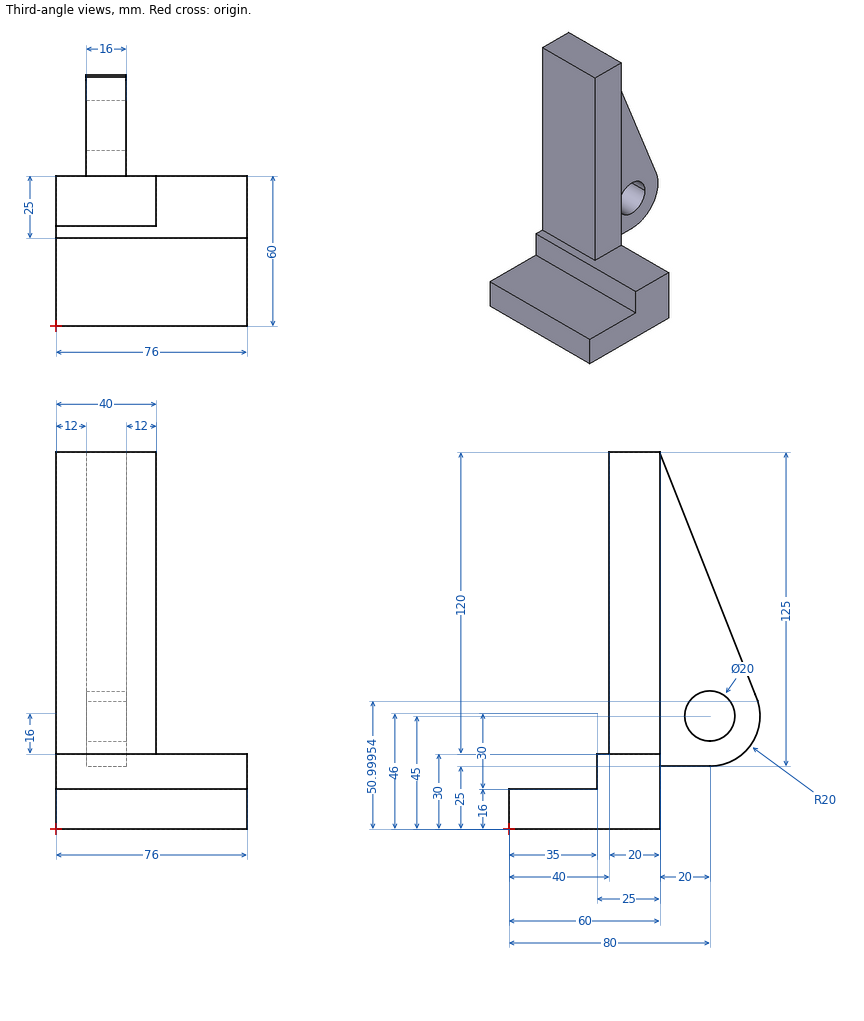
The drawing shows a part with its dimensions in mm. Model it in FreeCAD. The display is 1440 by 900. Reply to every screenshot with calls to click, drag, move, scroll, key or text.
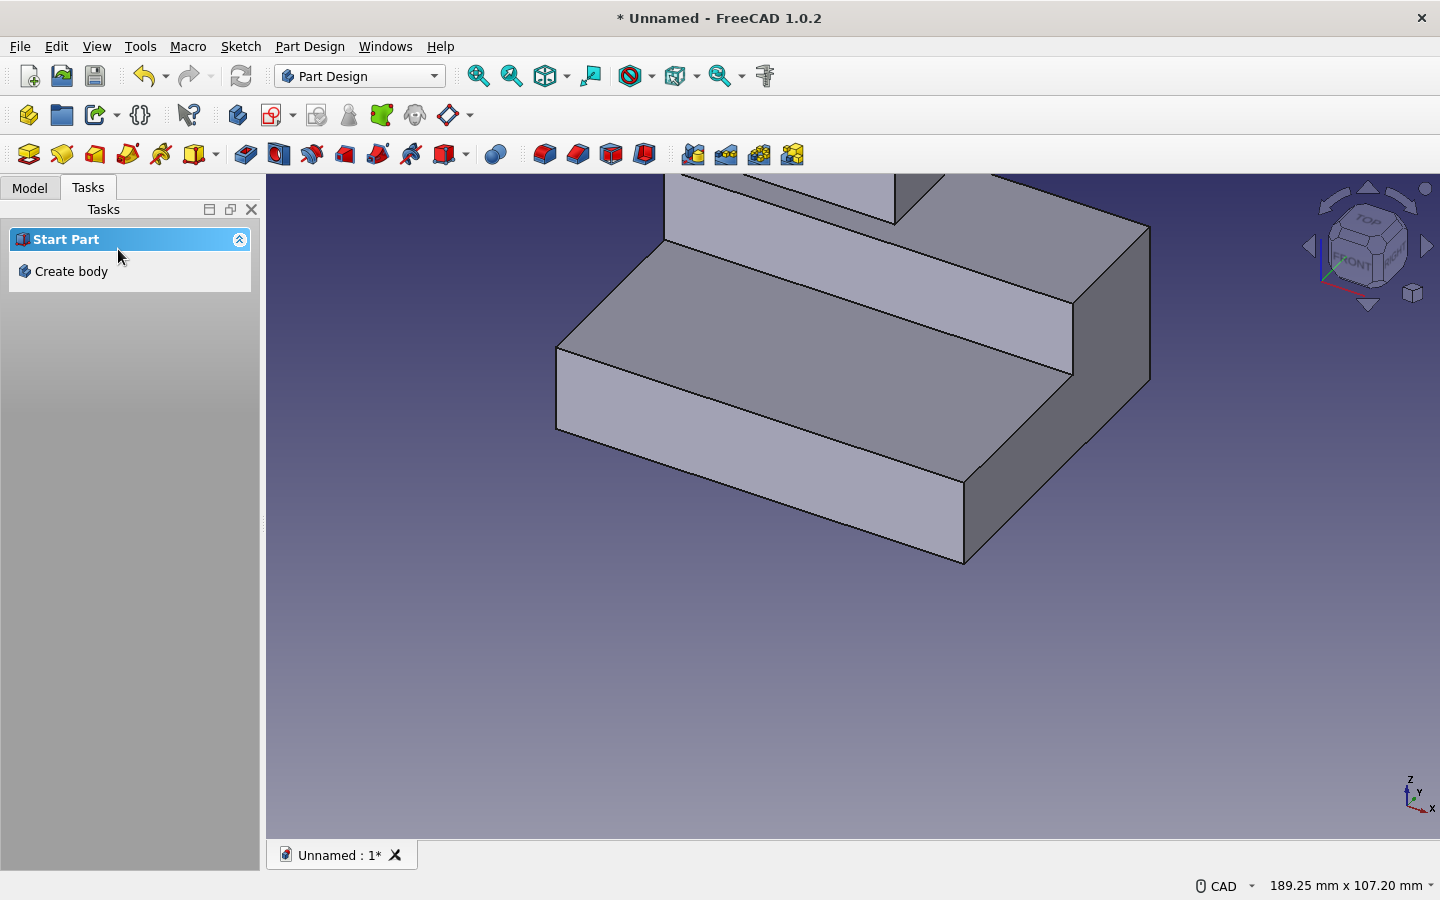
key(v)
key(f)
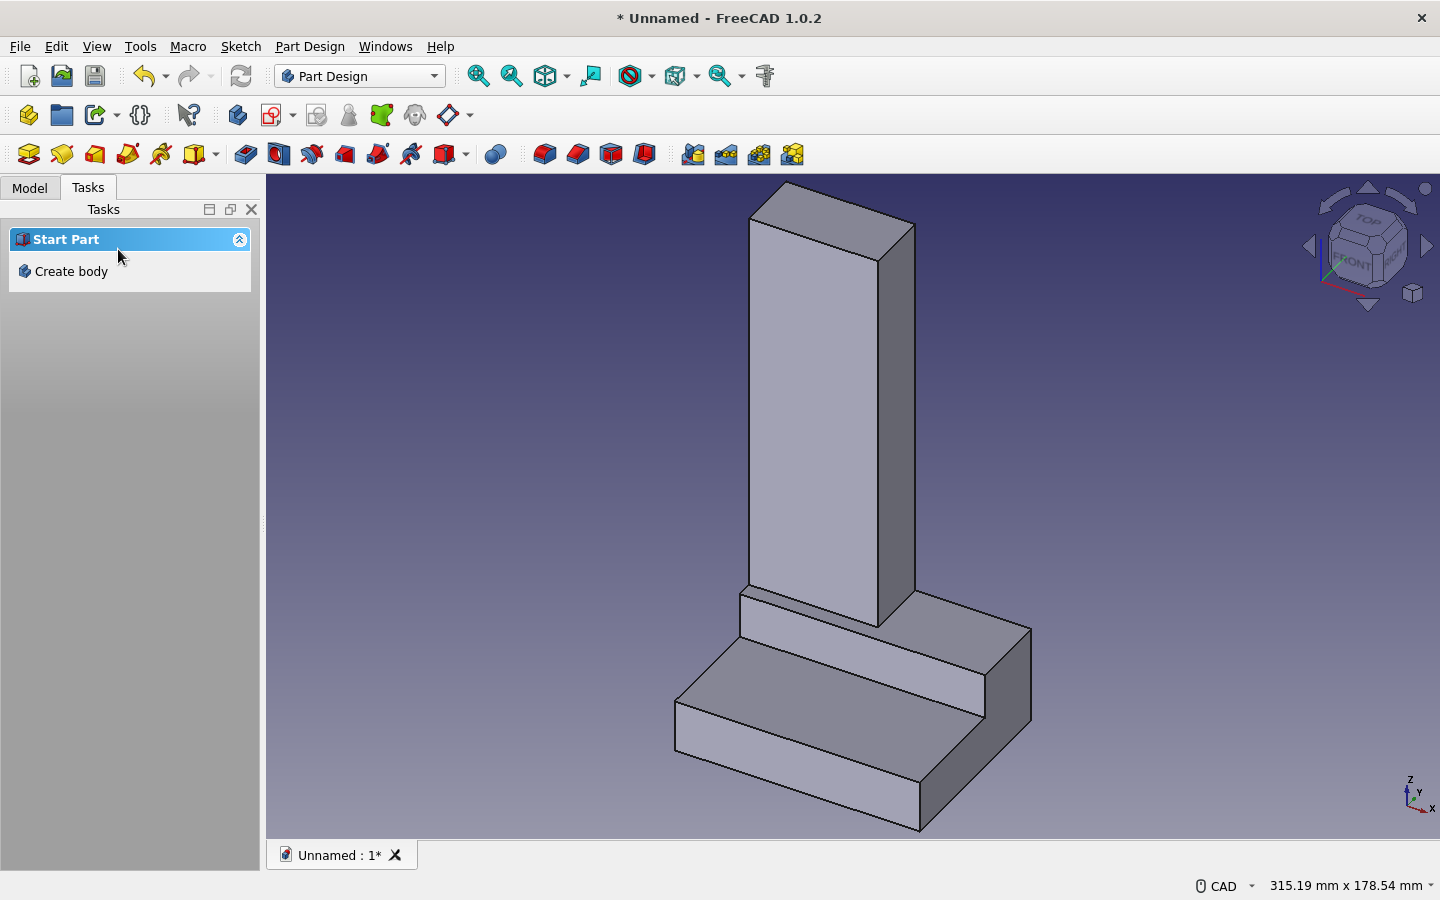
click(897, 320)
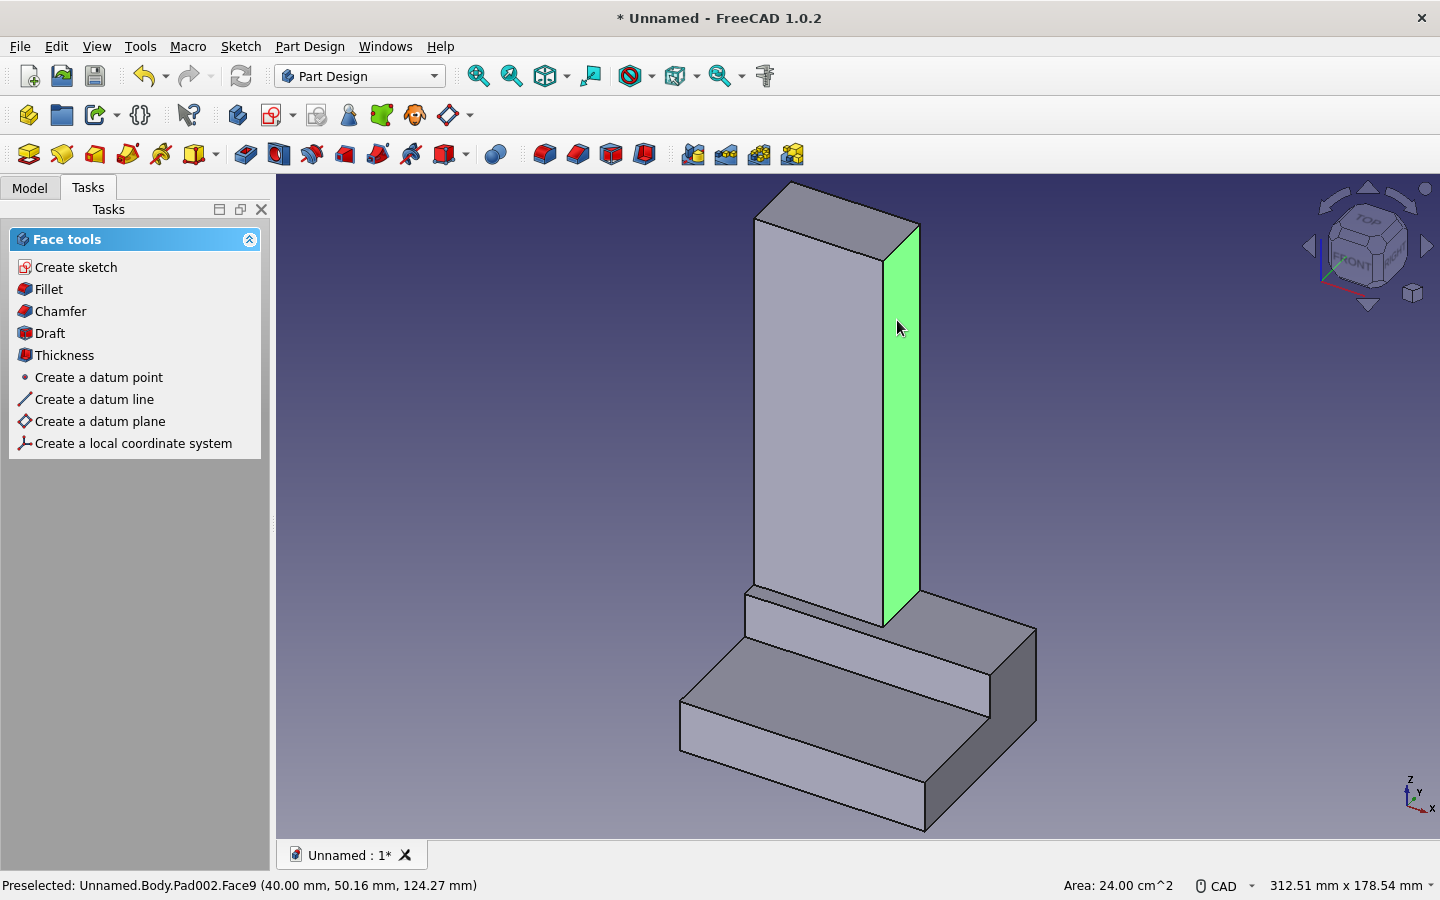
click(270, 116)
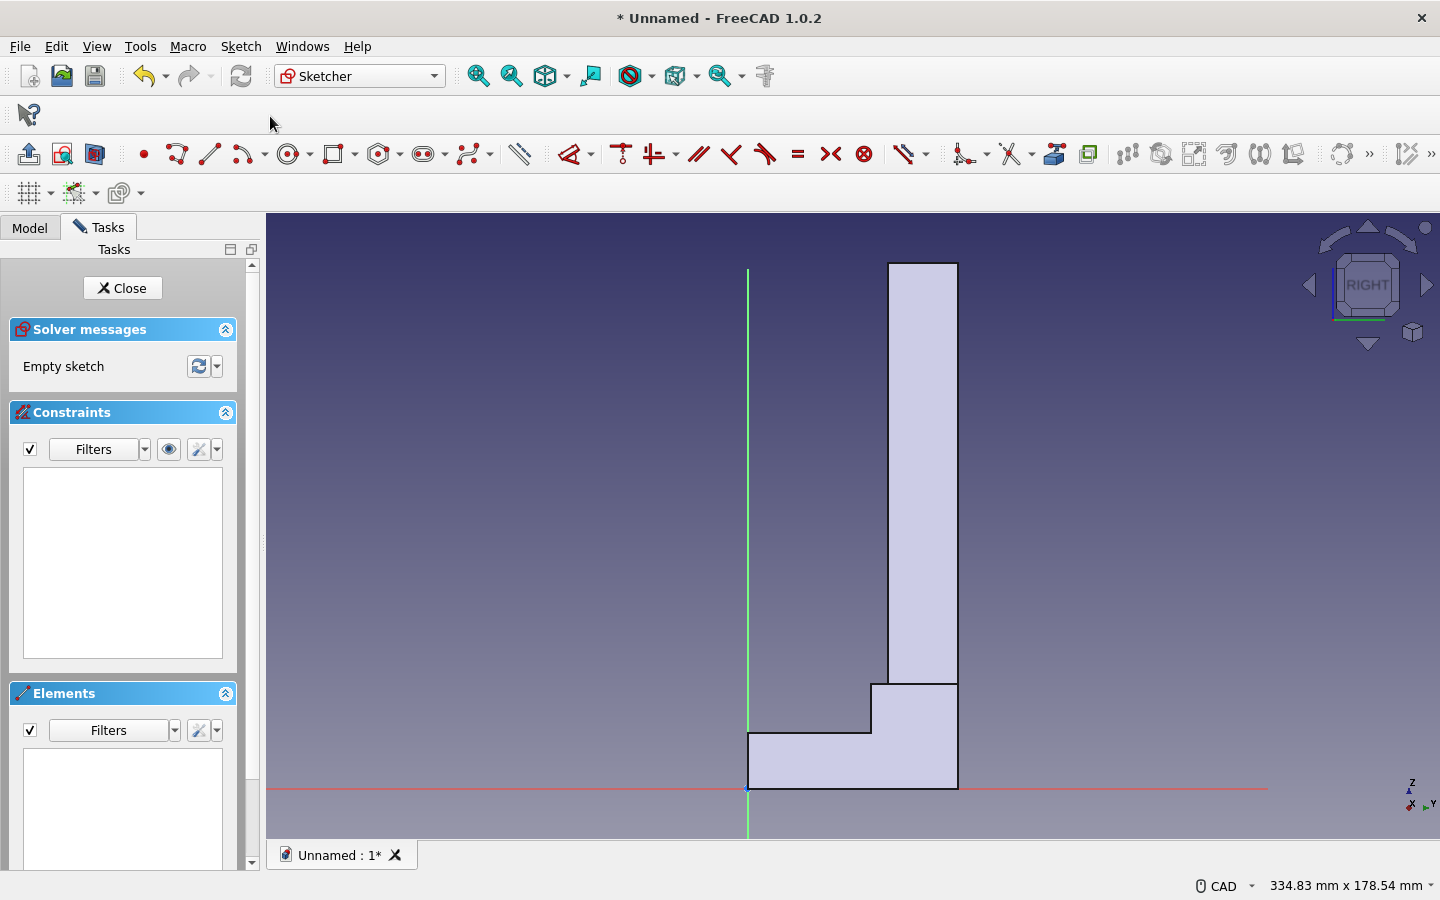
key(q)
key(s)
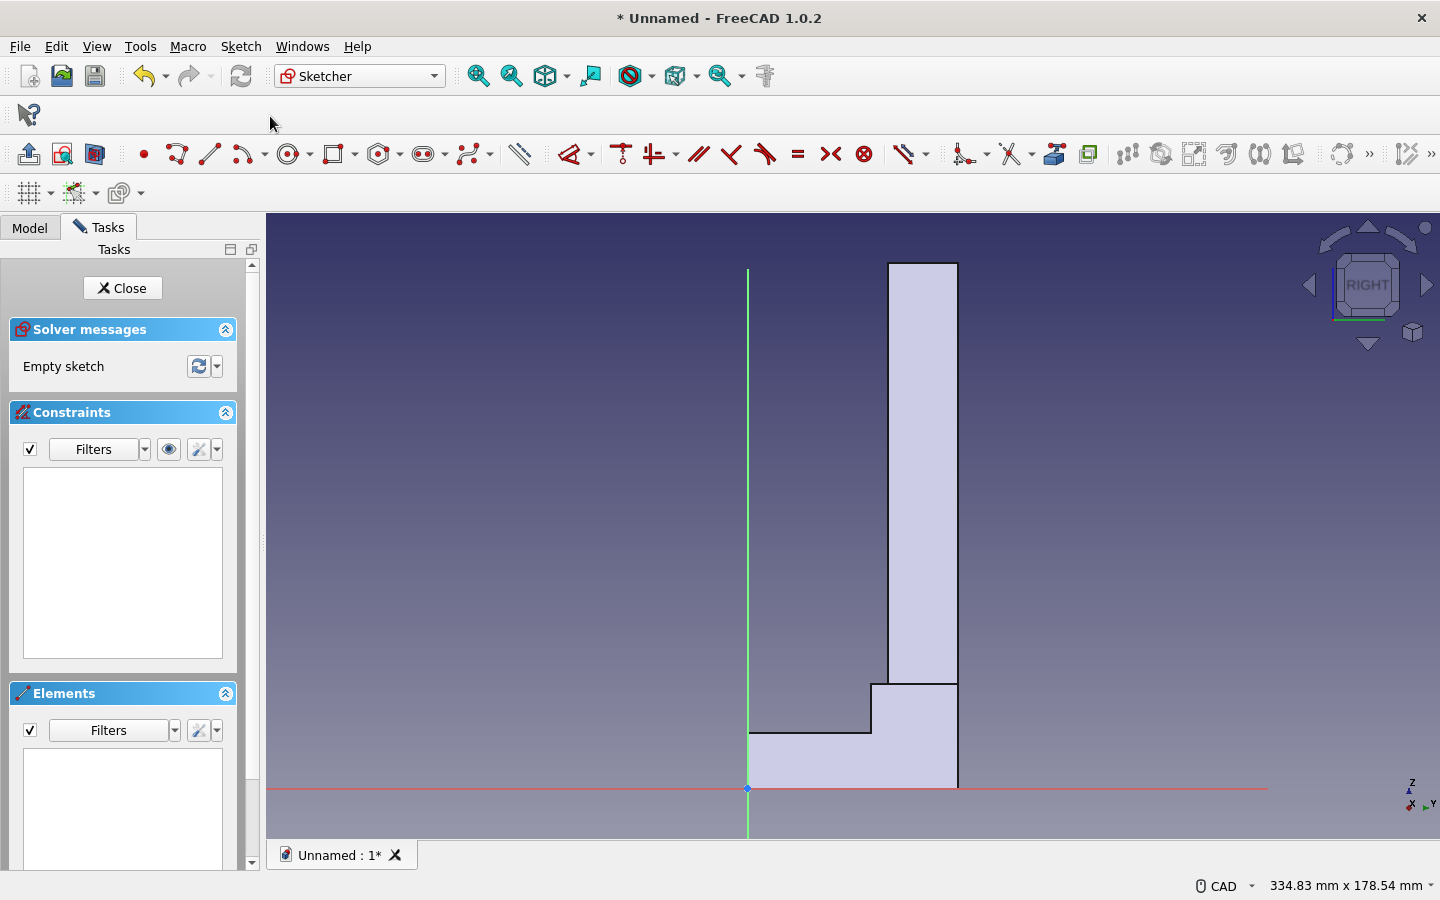
scroll(294, 526, down, 1)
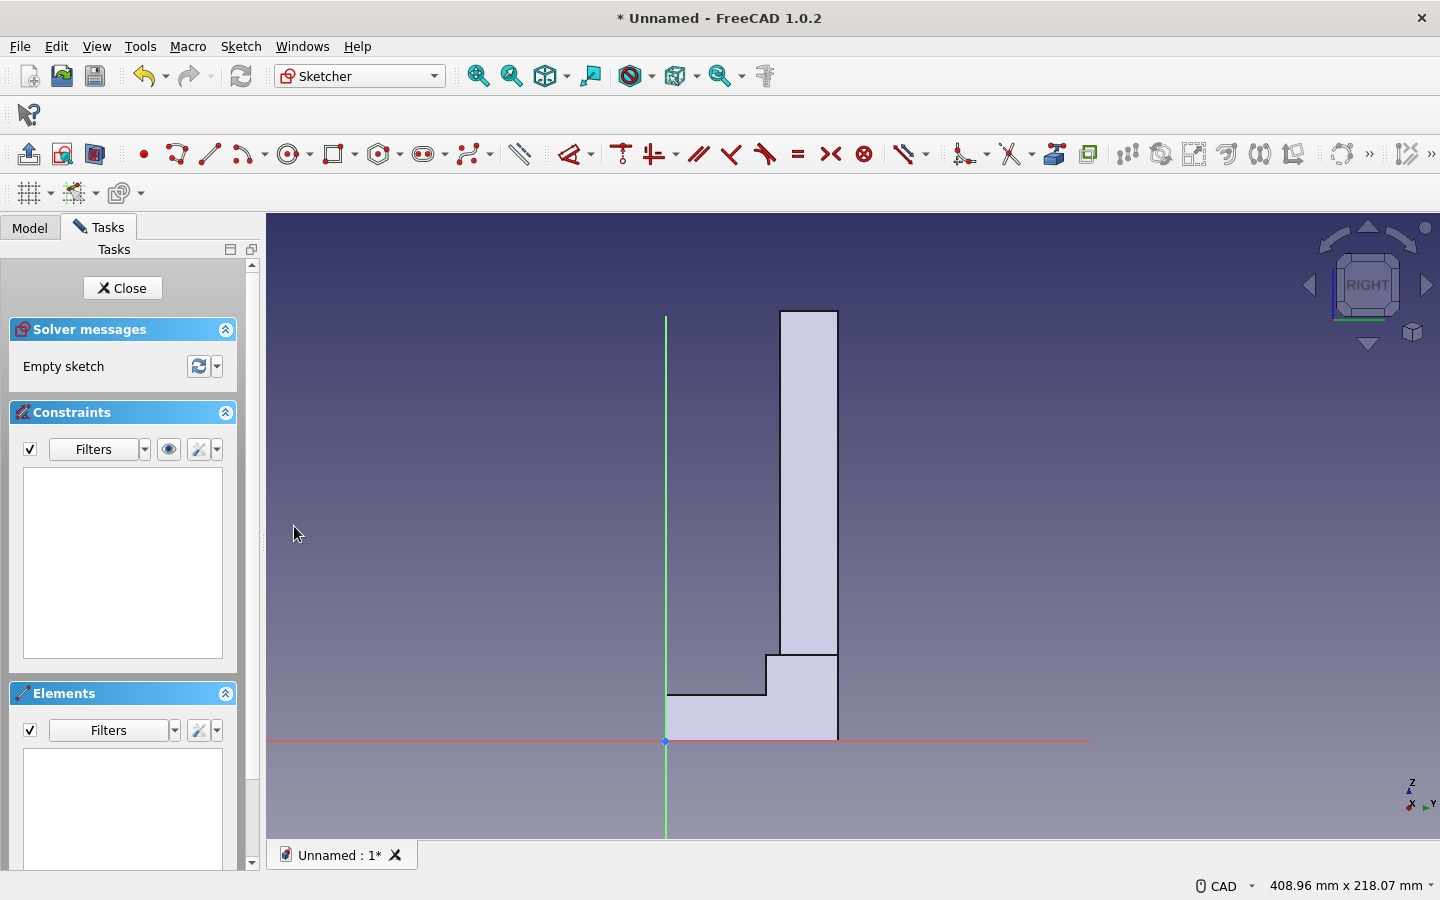
click(177, 154)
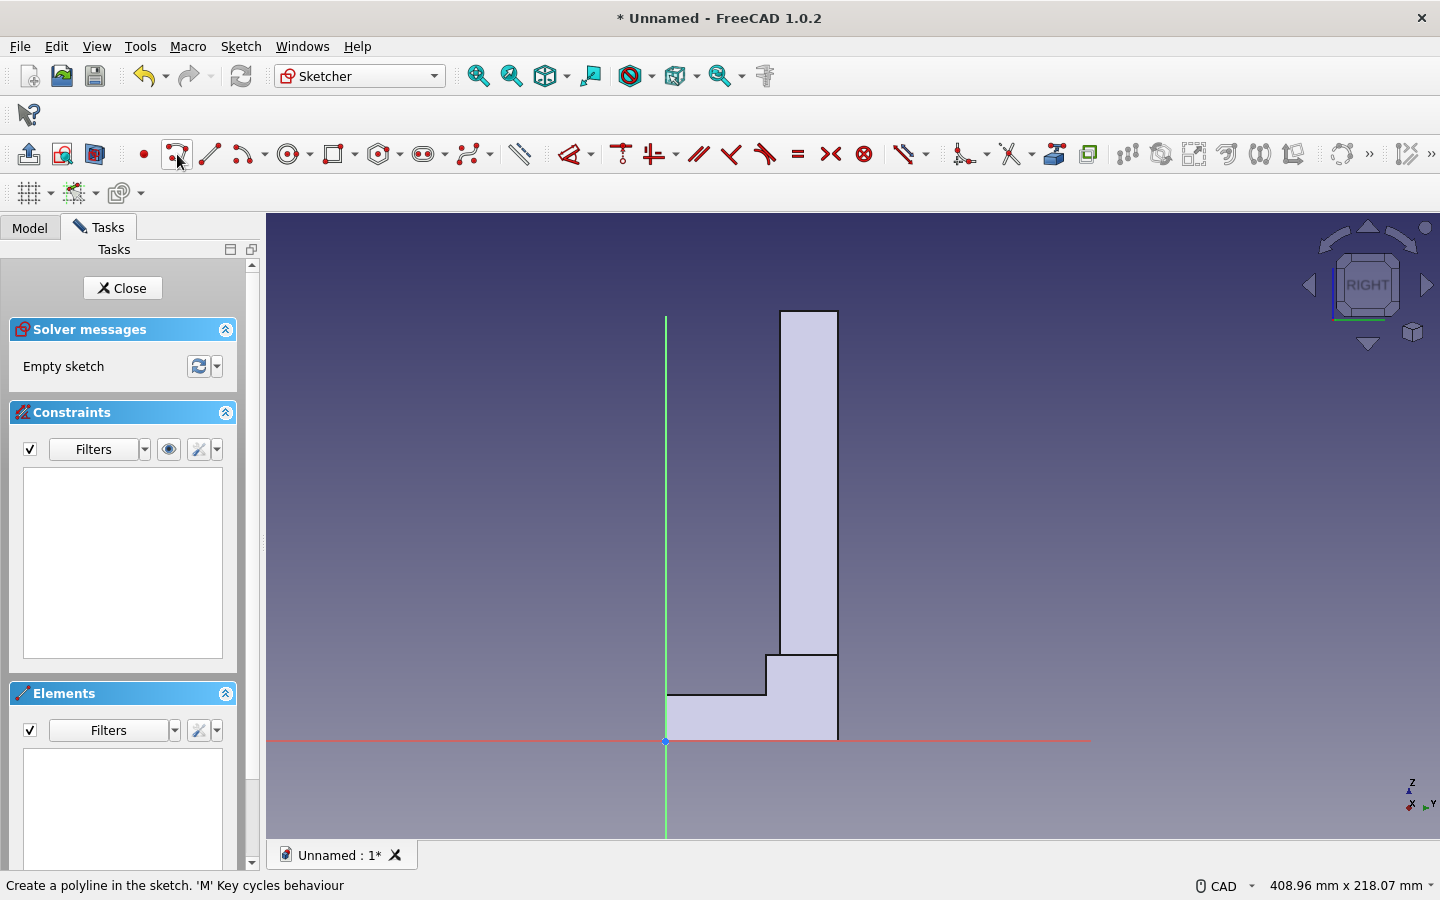
click(950, 595)
click(838, 311)
click(838, 670)
click(895, 670)
right_click(895, 670)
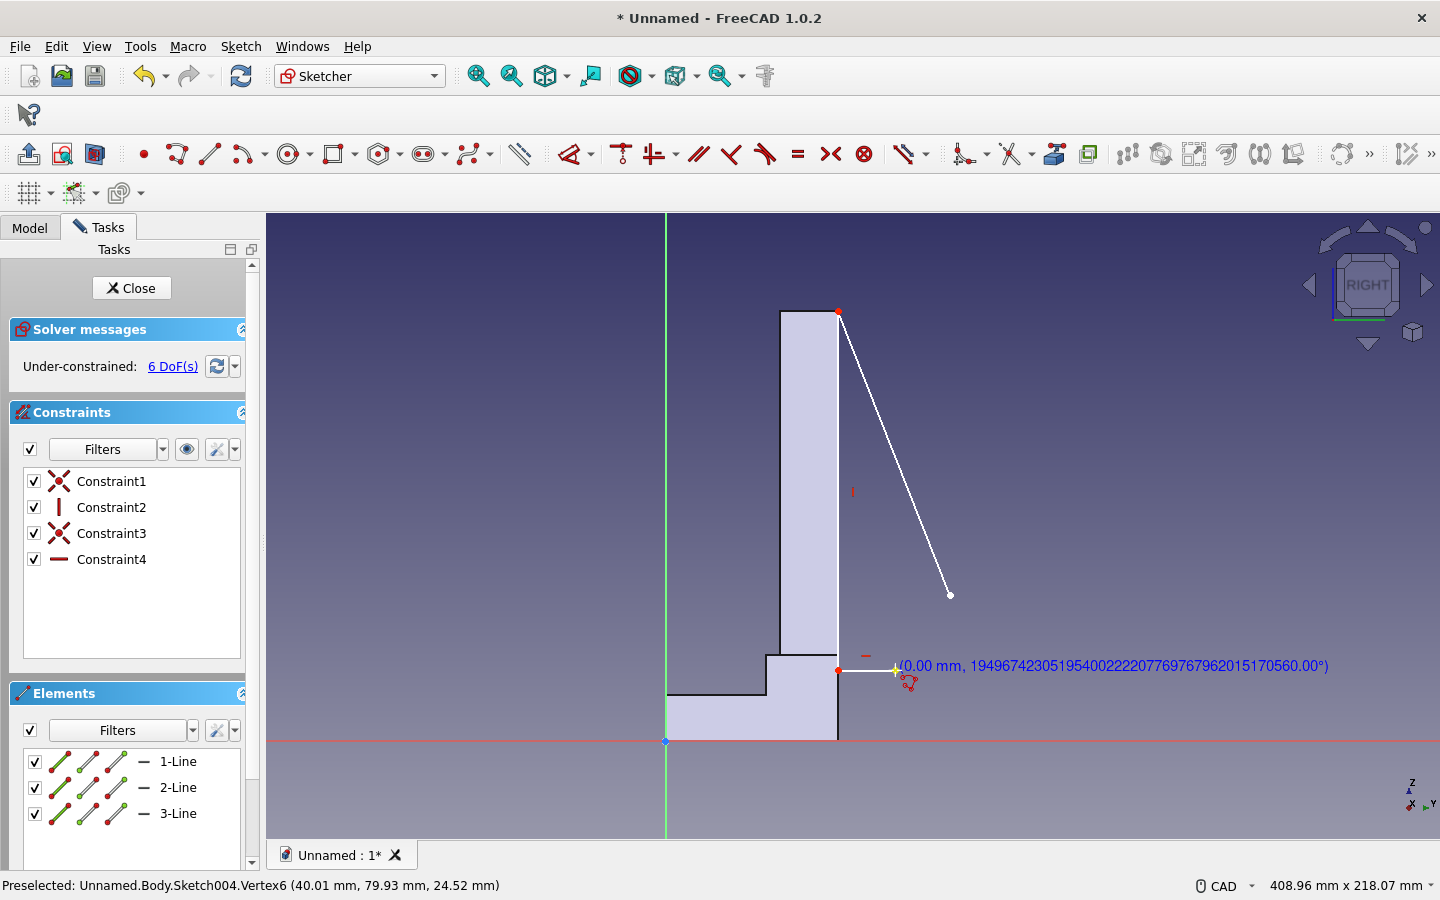
key(g)
key(3)
key(a)